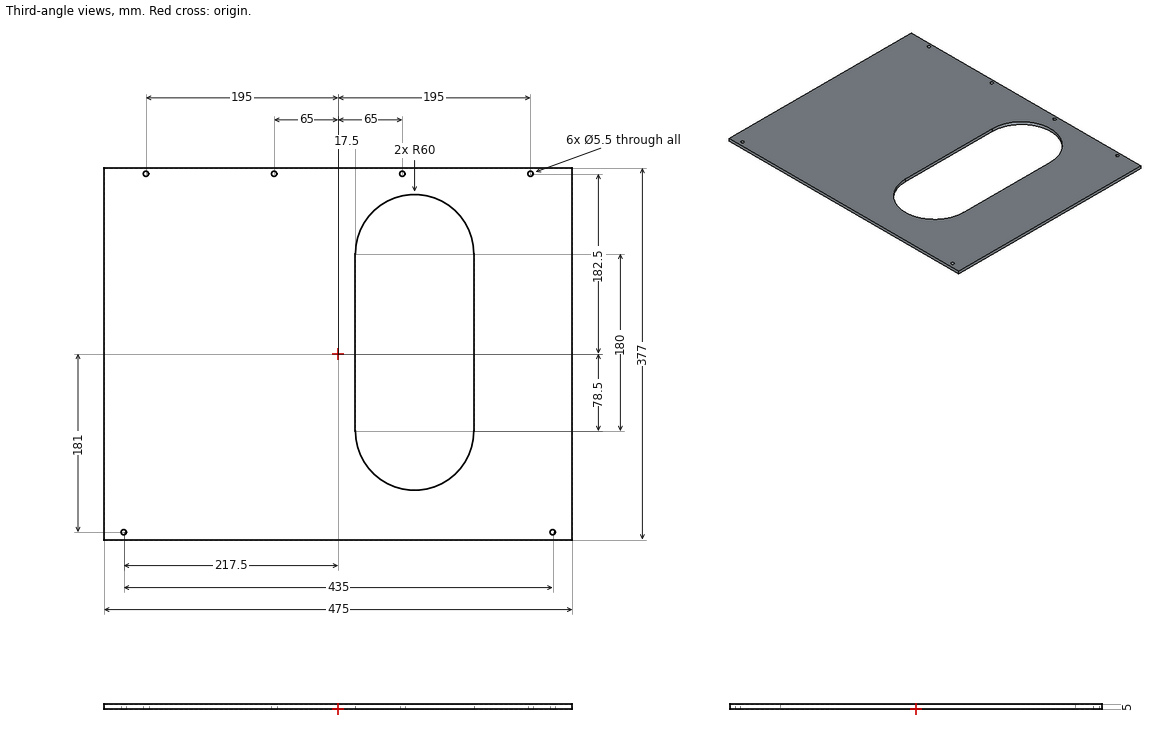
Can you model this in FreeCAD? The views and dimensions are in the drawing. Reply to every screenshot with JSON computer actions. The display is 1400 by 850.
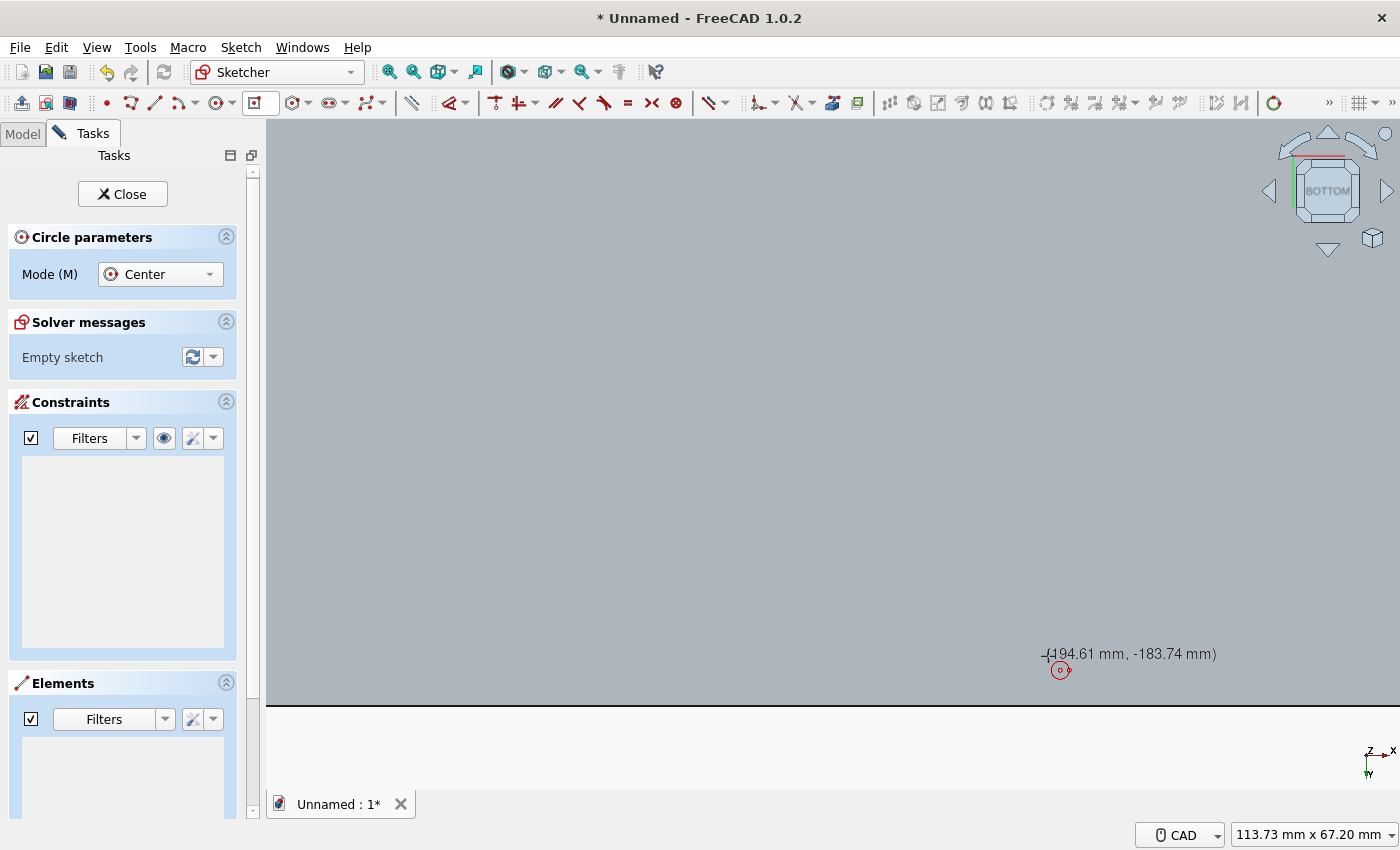
{"action": "scroll", "coordinate": [972, 656], "scroll_direction": "down", "scroll_amount": 11}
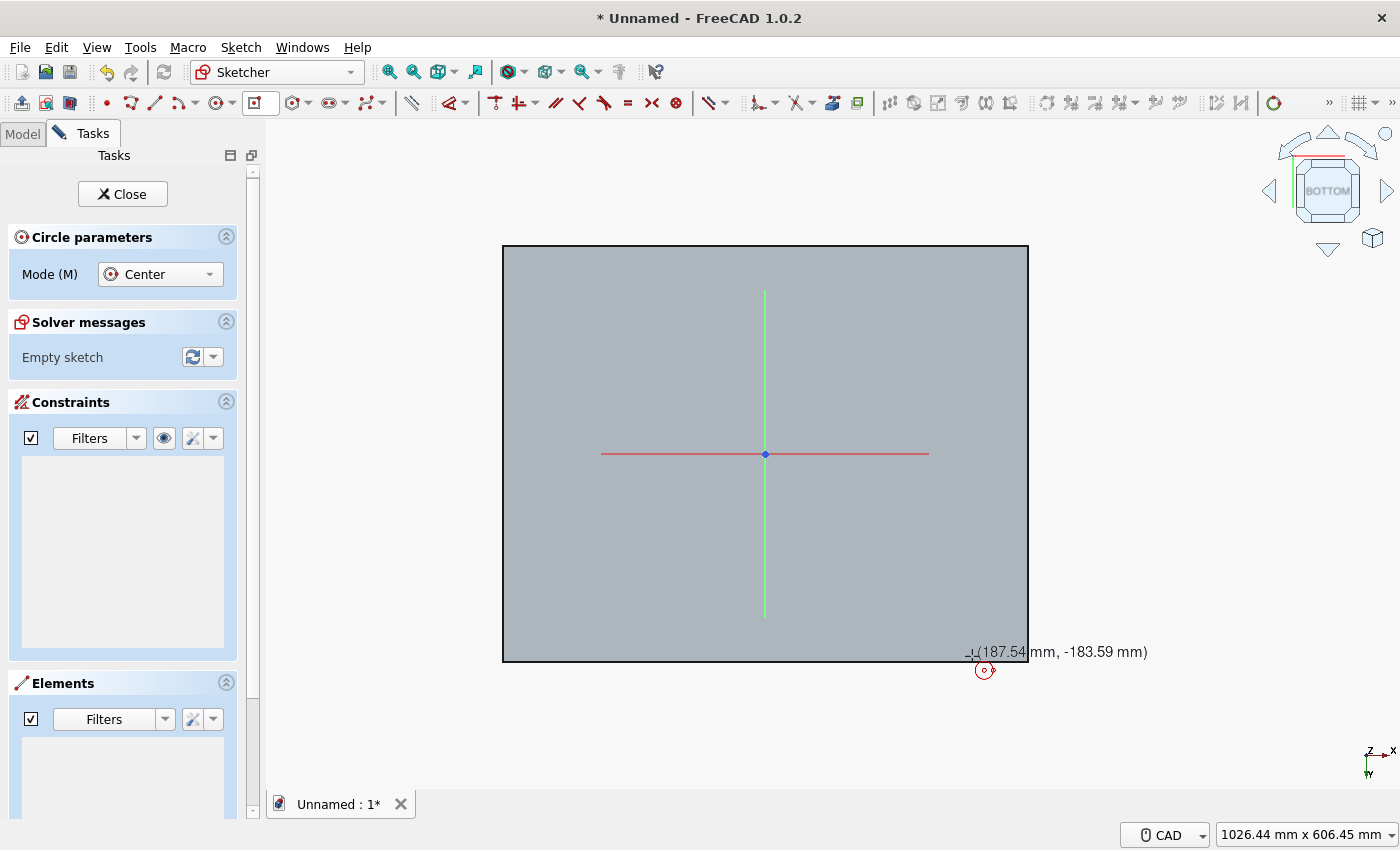
{"action": "left_click", "coordinate": [981, 656]}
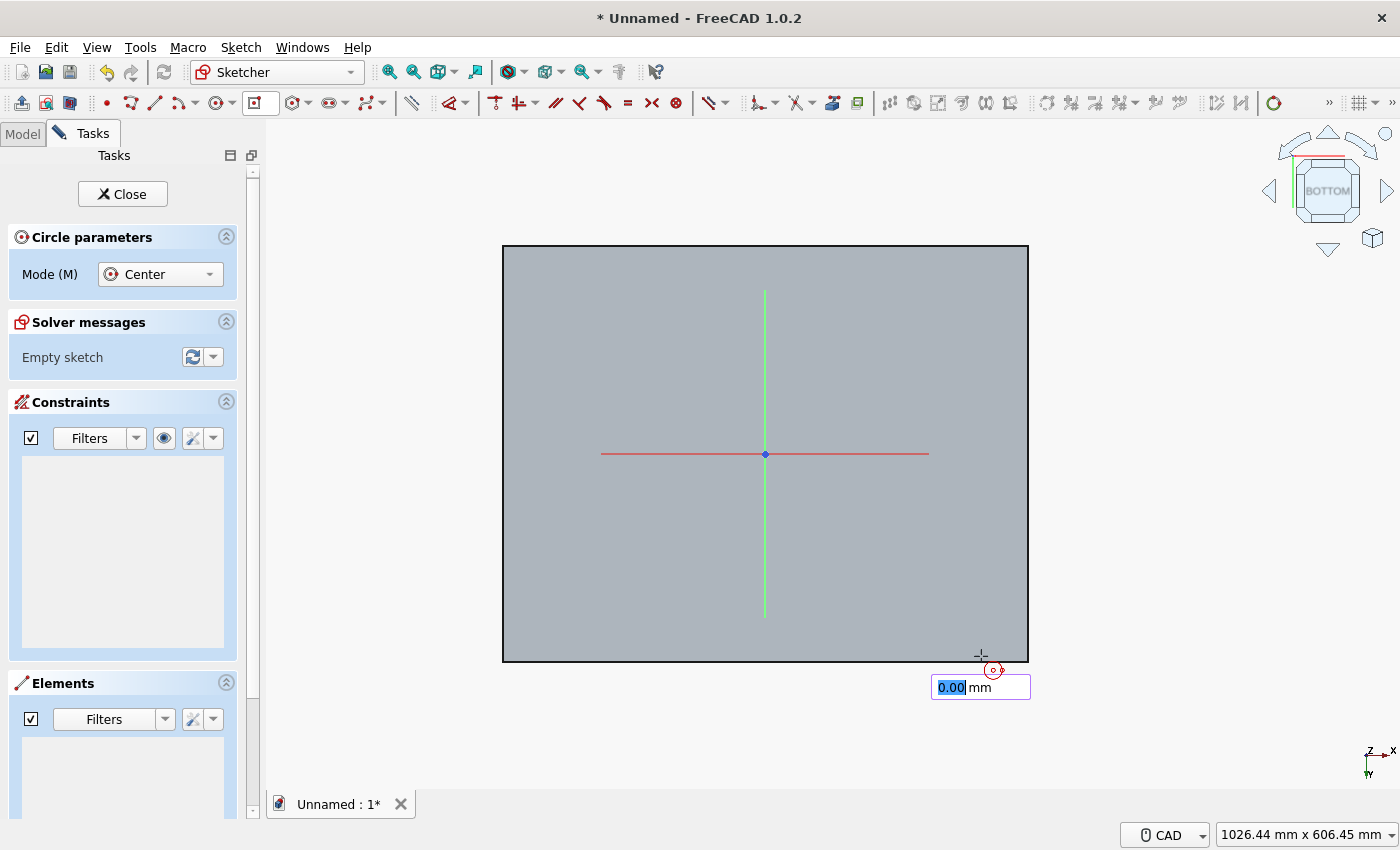
{"action": "scroll", "coordinate": [983, 653], "scroll_direction": "up", "scroll_amount": 9}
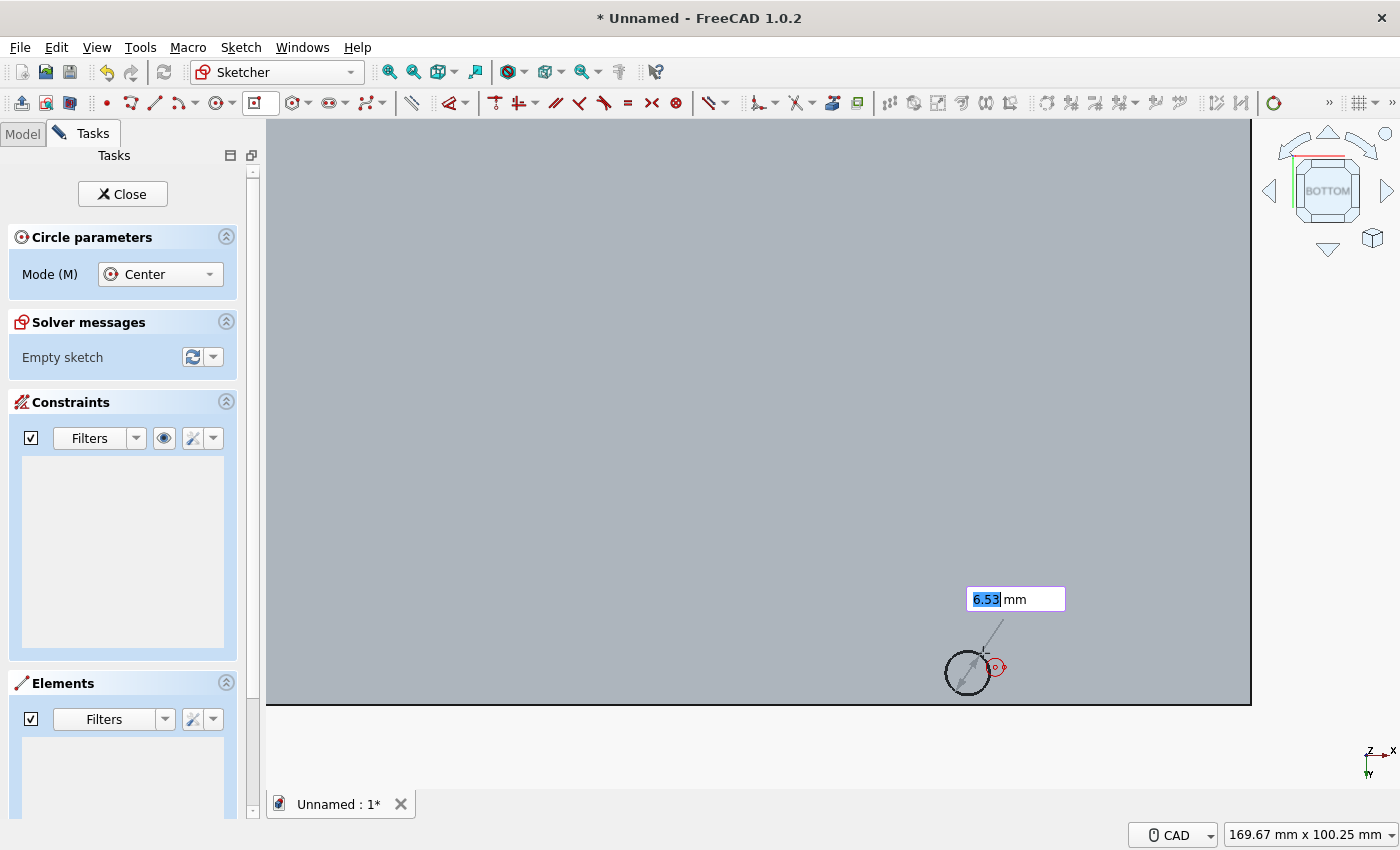
{"action": "left_click", "coordinate": [979, 652]}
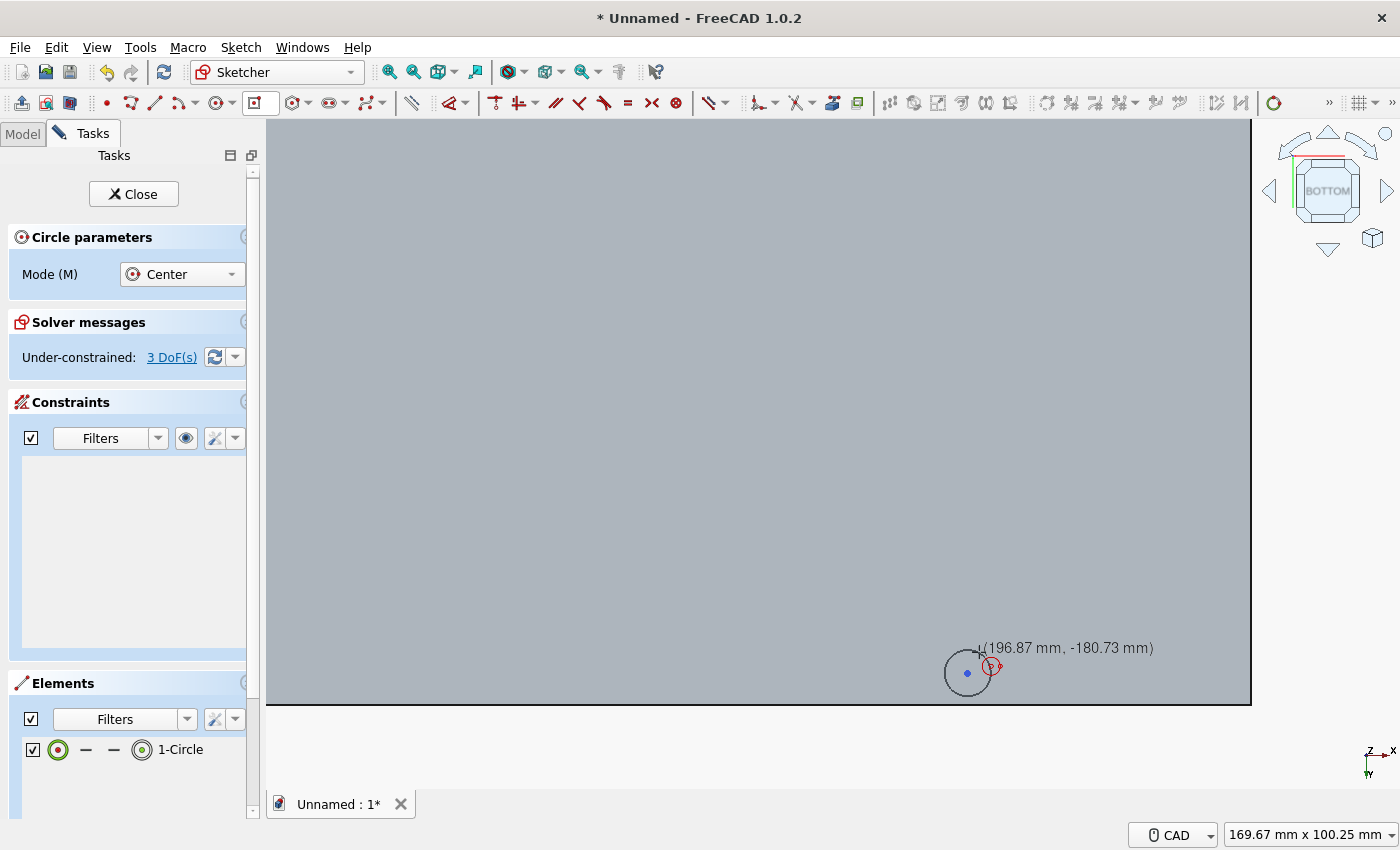
{"action": "scroll", "coordinate": [983, 653], "scroll_direction": "down", "scroll_amount": 9}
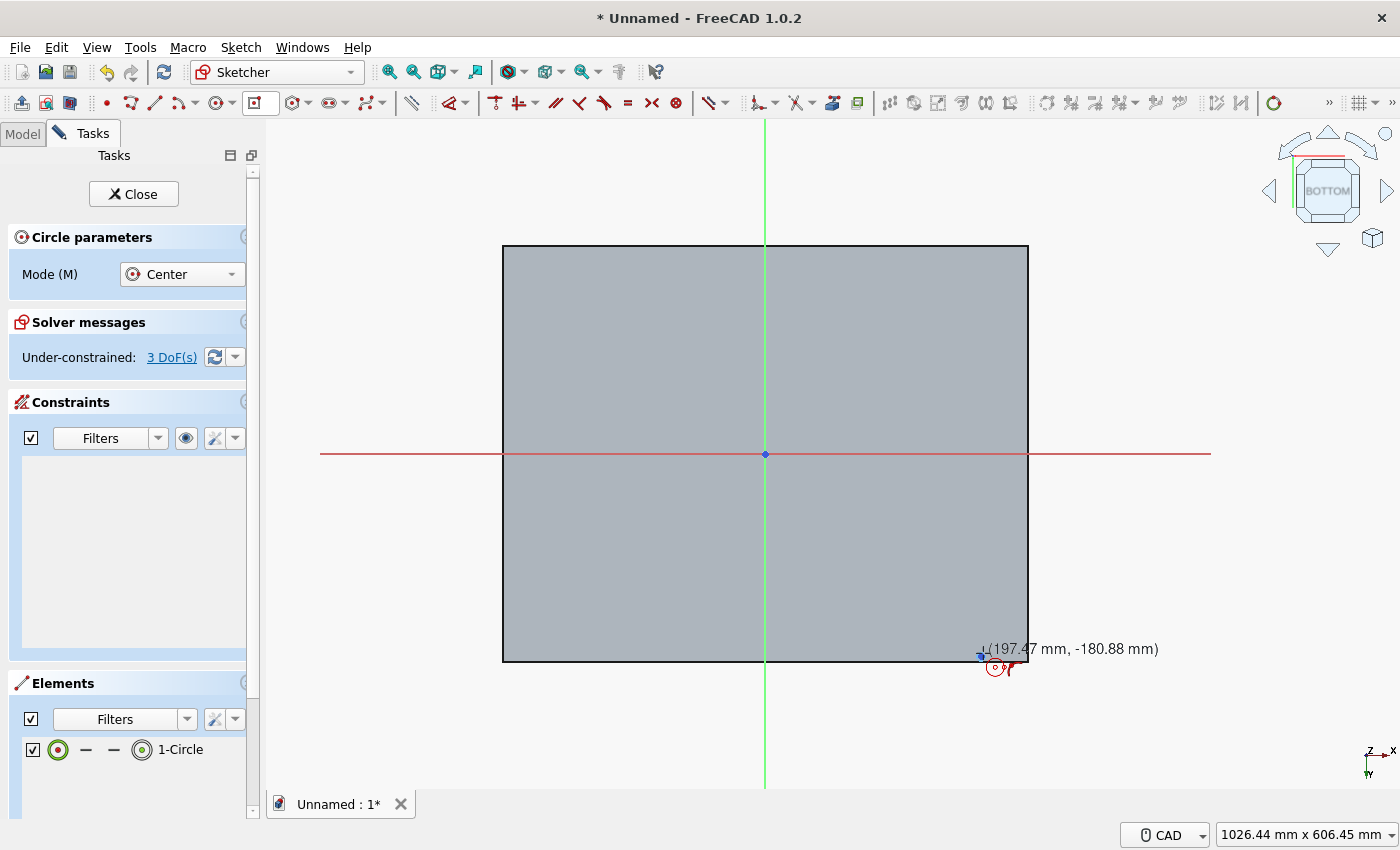
{"action": "scroll", "coordinate": [837, 656], "scroll_direction": "up", "scroll_amount": 11}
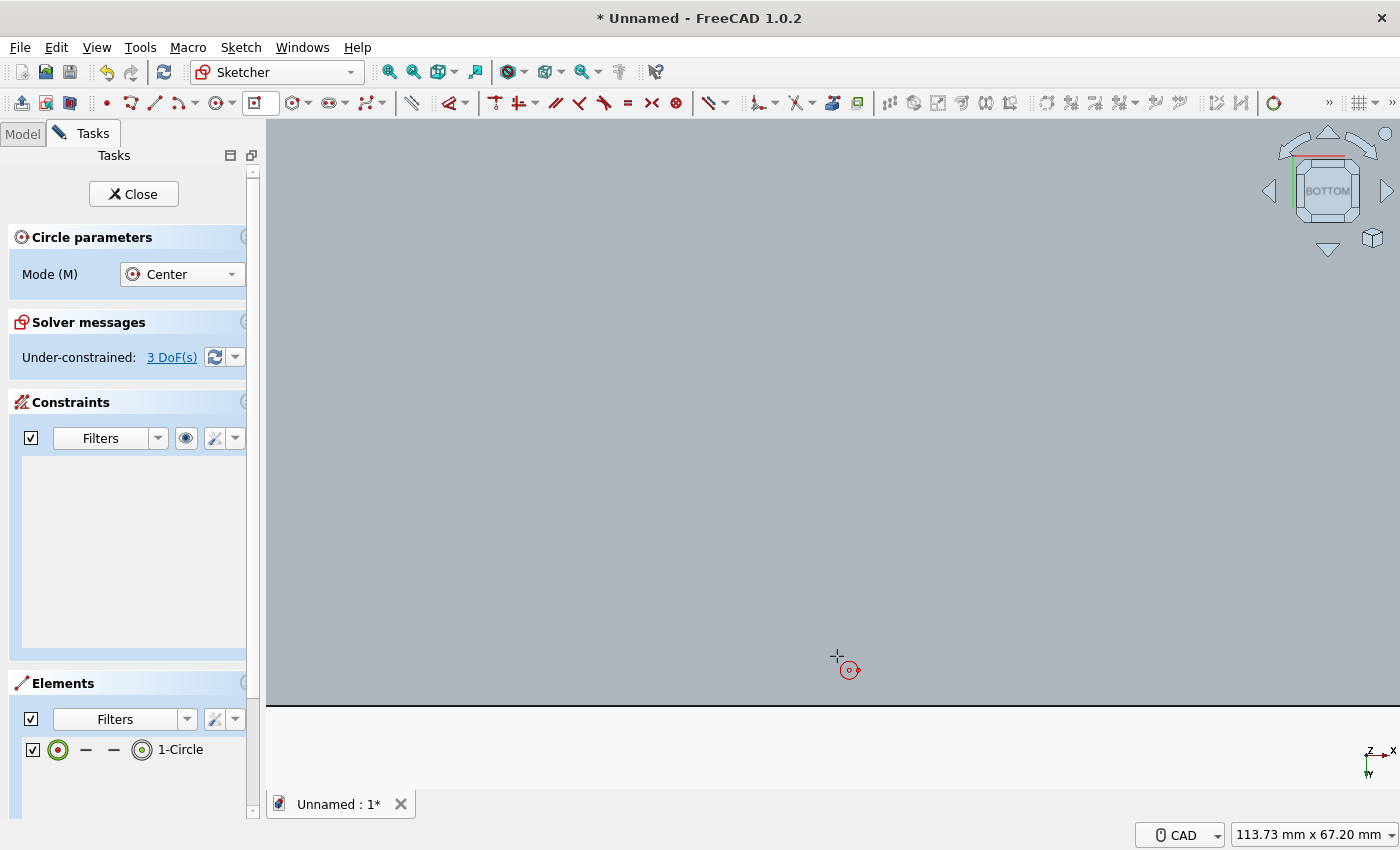
{"action": "scroll", "coordinate": [837, 656], "scroll_direction": "down", "scroll_amount": 11}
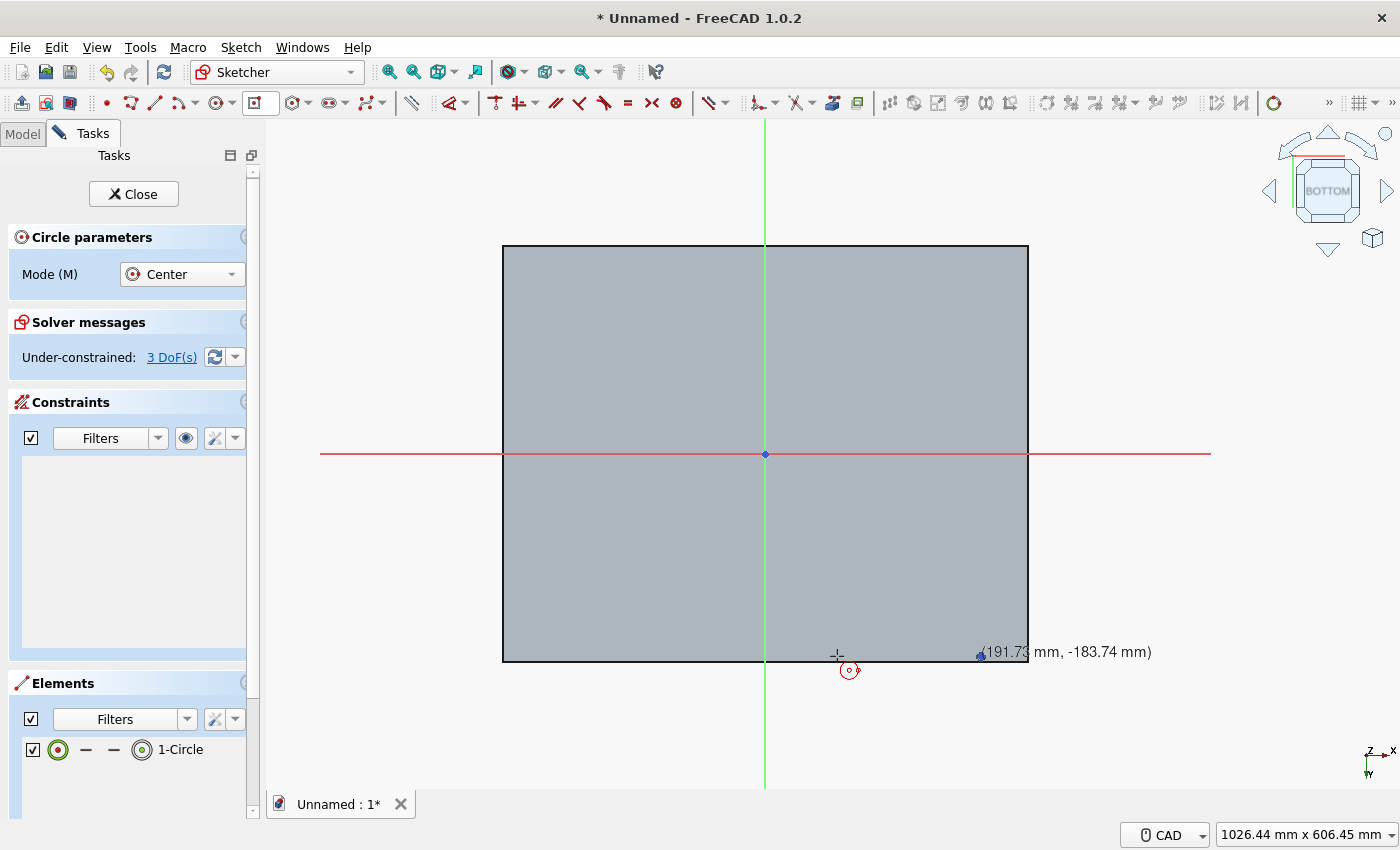
{"action": "left_click", "coordinate": [837, 656]}